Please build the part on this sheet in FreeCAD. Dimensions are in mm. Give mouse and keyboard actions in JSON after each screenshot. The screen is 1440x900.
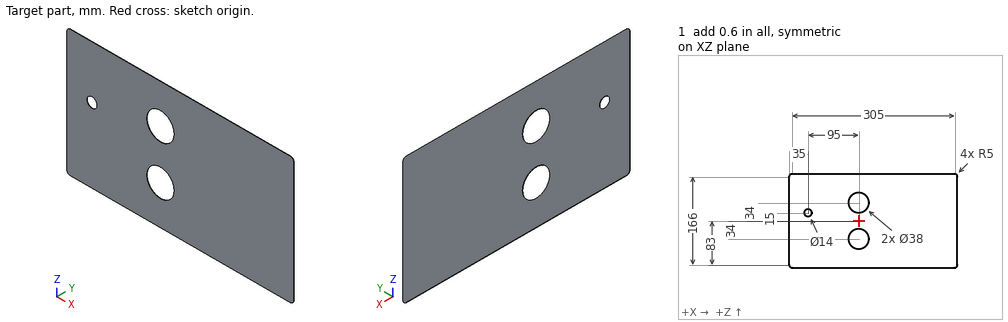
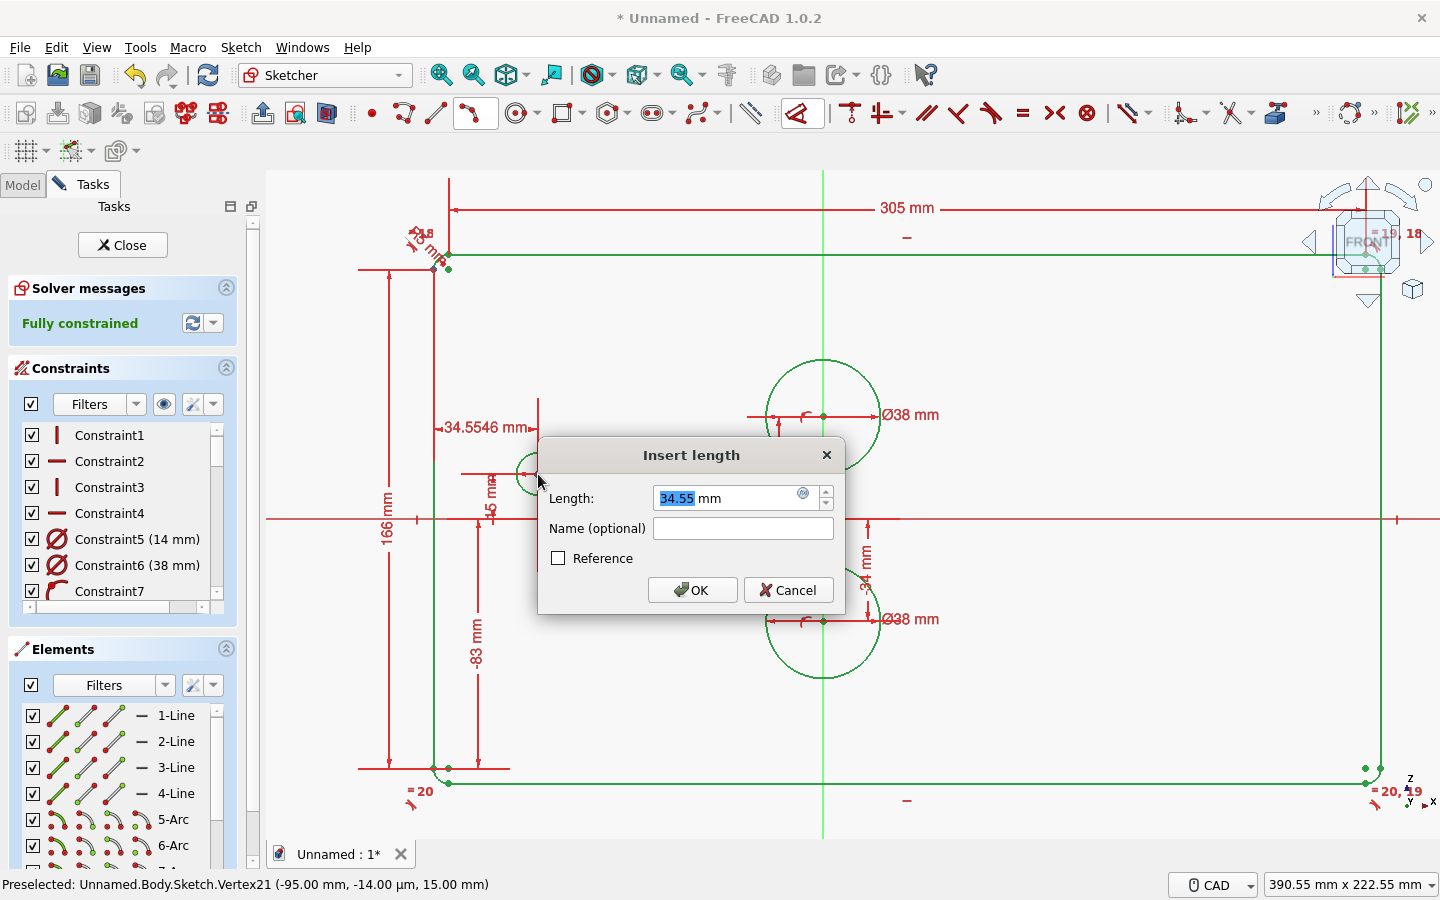
{"action": "type", "text": "35"}
{"action": "key", "text": "Return"}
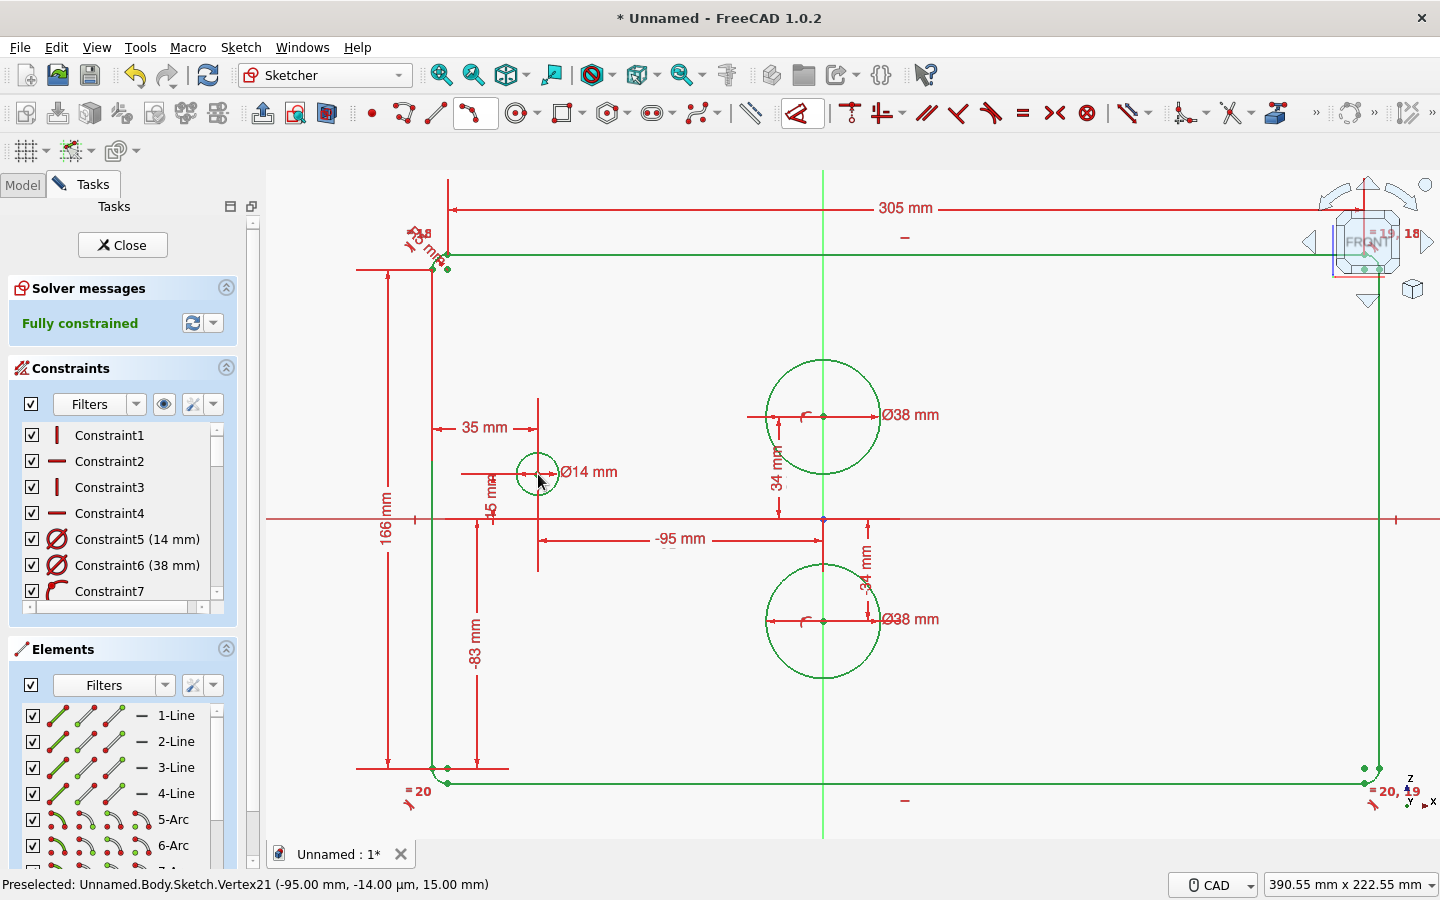
{"action": "left_click", "coordinate": [123, 245]}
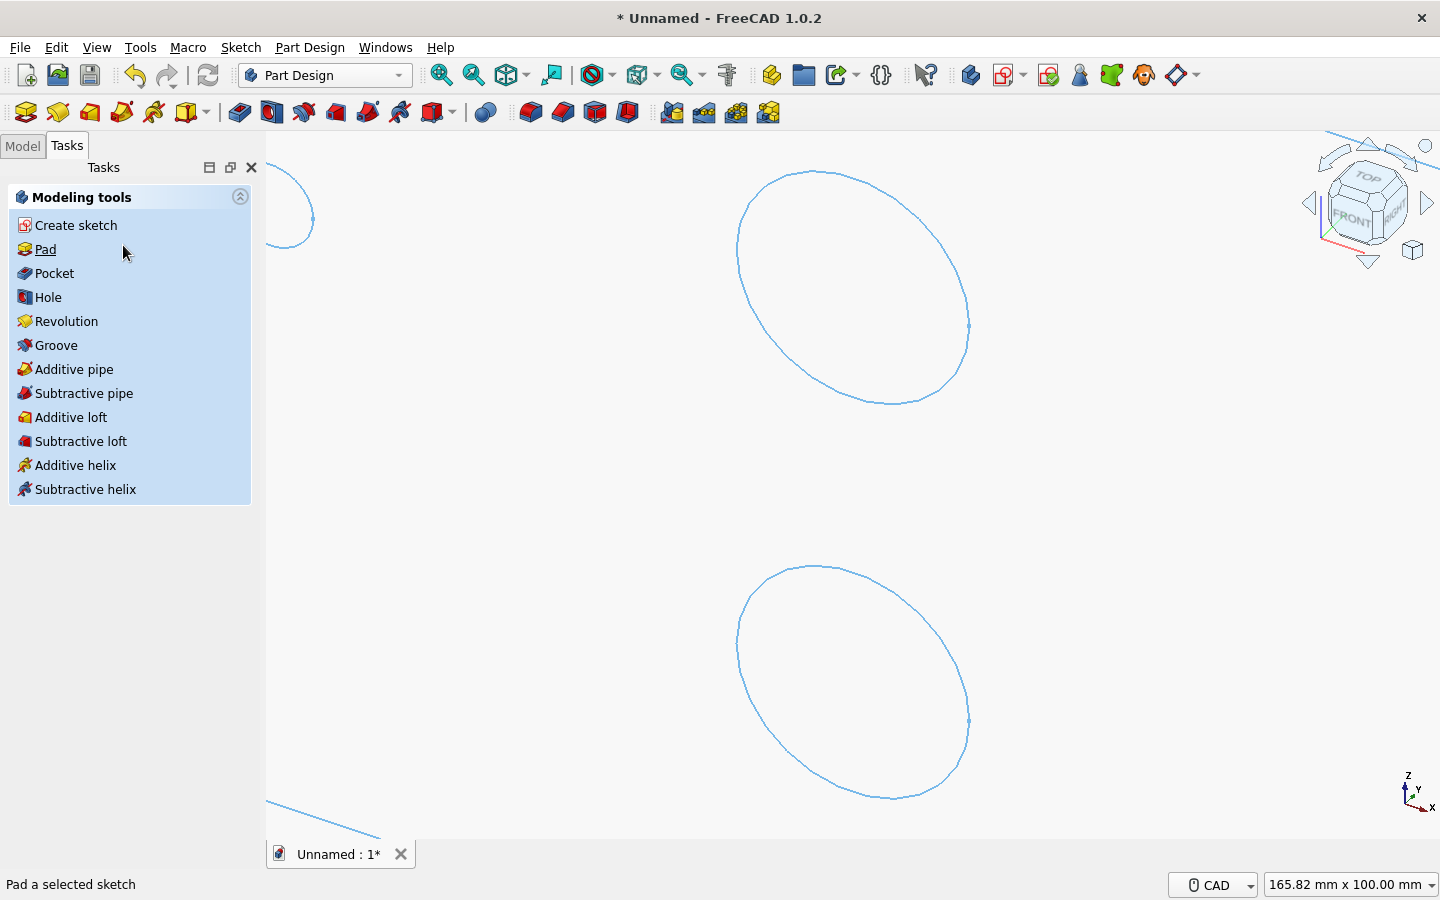
{"action": "left_click", "coordinate": [26, 112]}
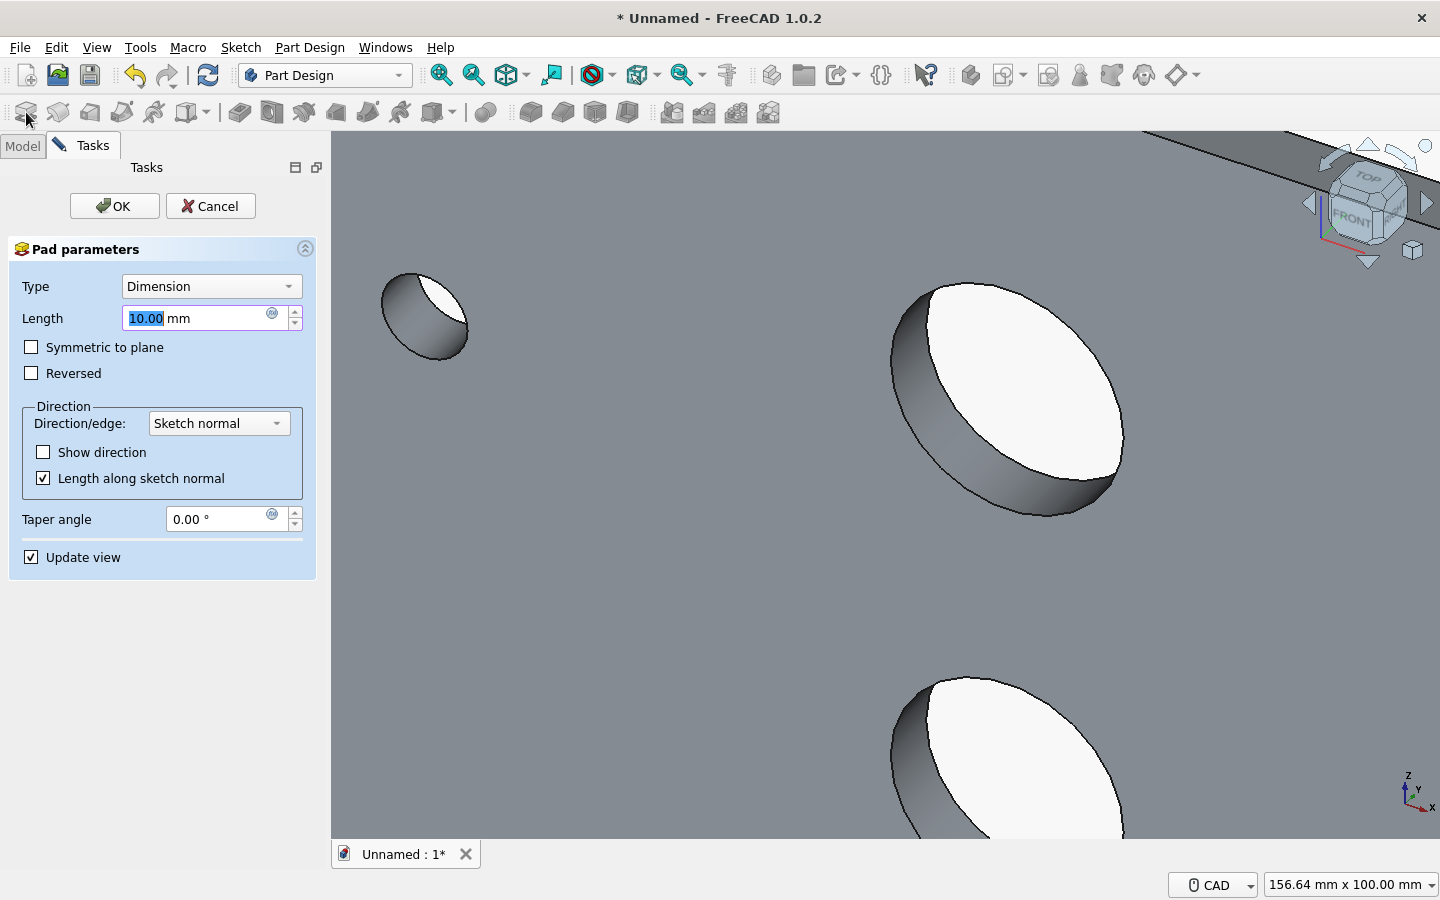
{"action": "type", "text": "0.6"}
{"action": "key", "text": "Tab"}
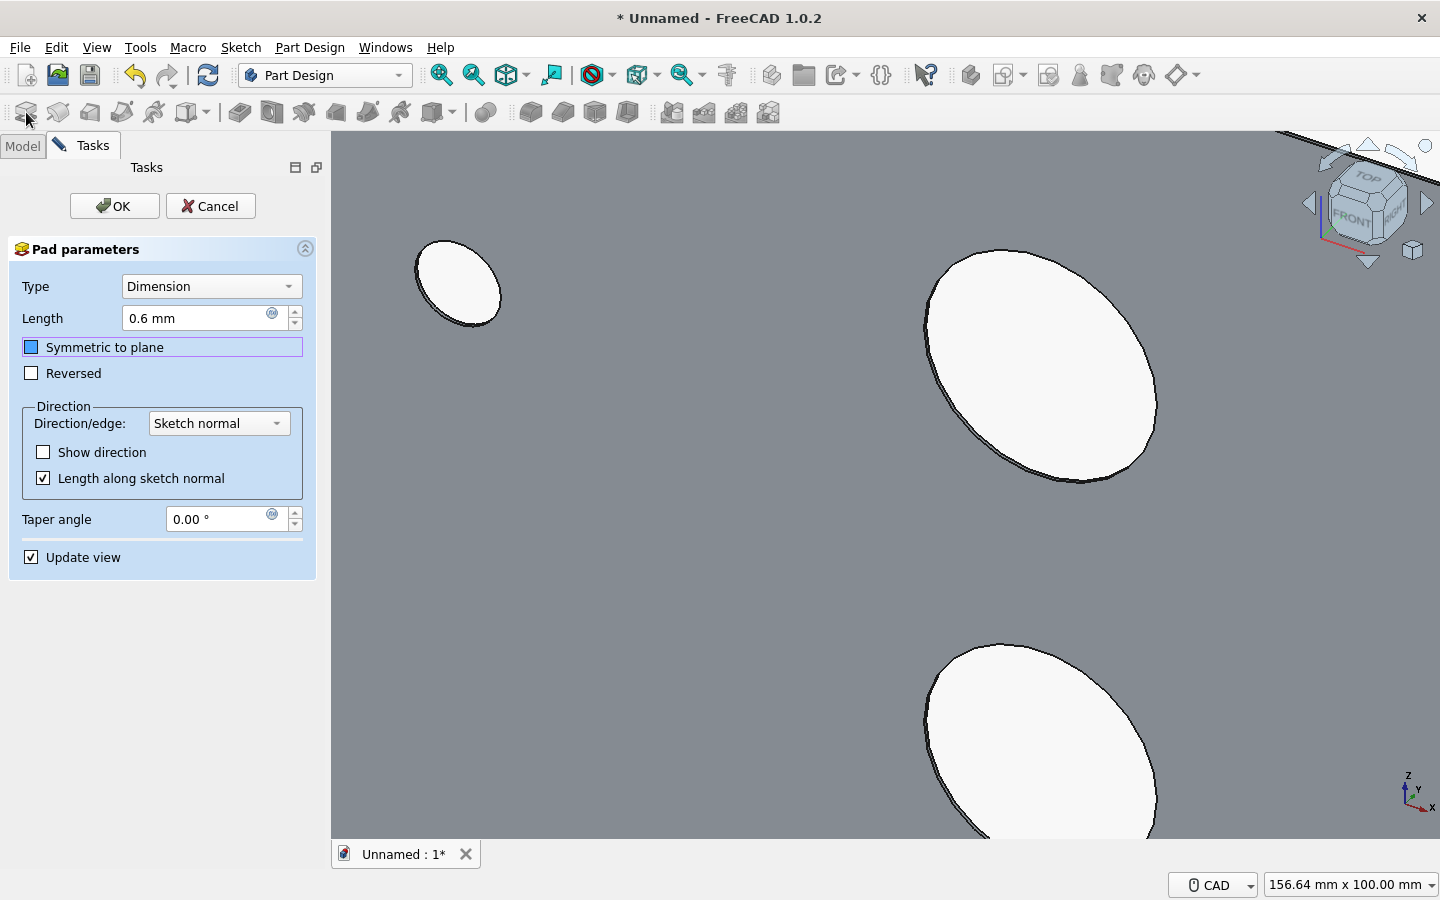
{"action": "left_click", "coordinate": [30, 347]}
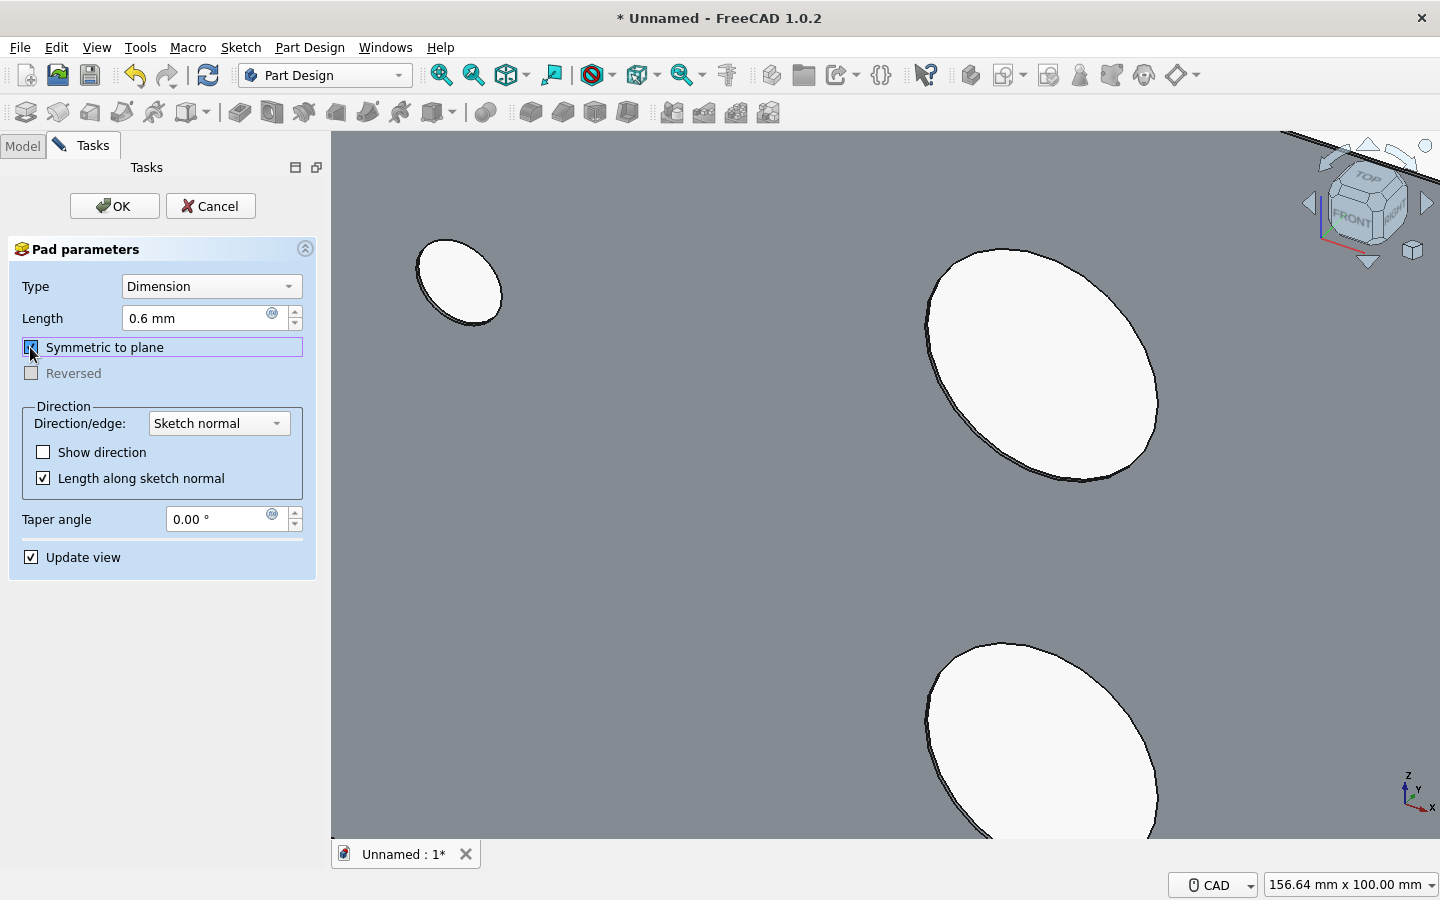
{"action": "left_click", "coordinate": [115, 206]}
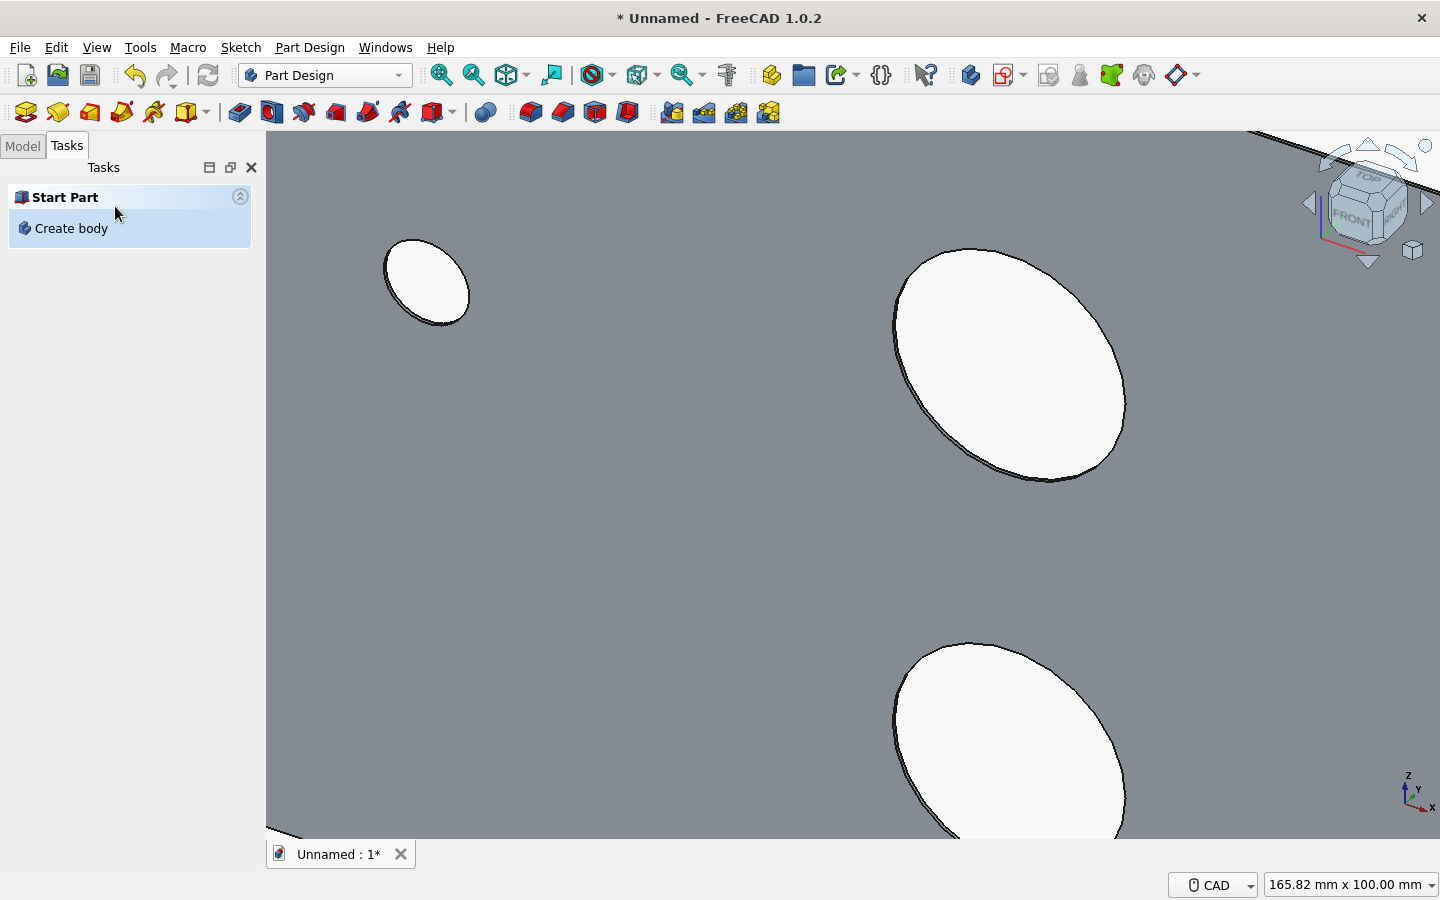
{"action": "key", "text": "0"}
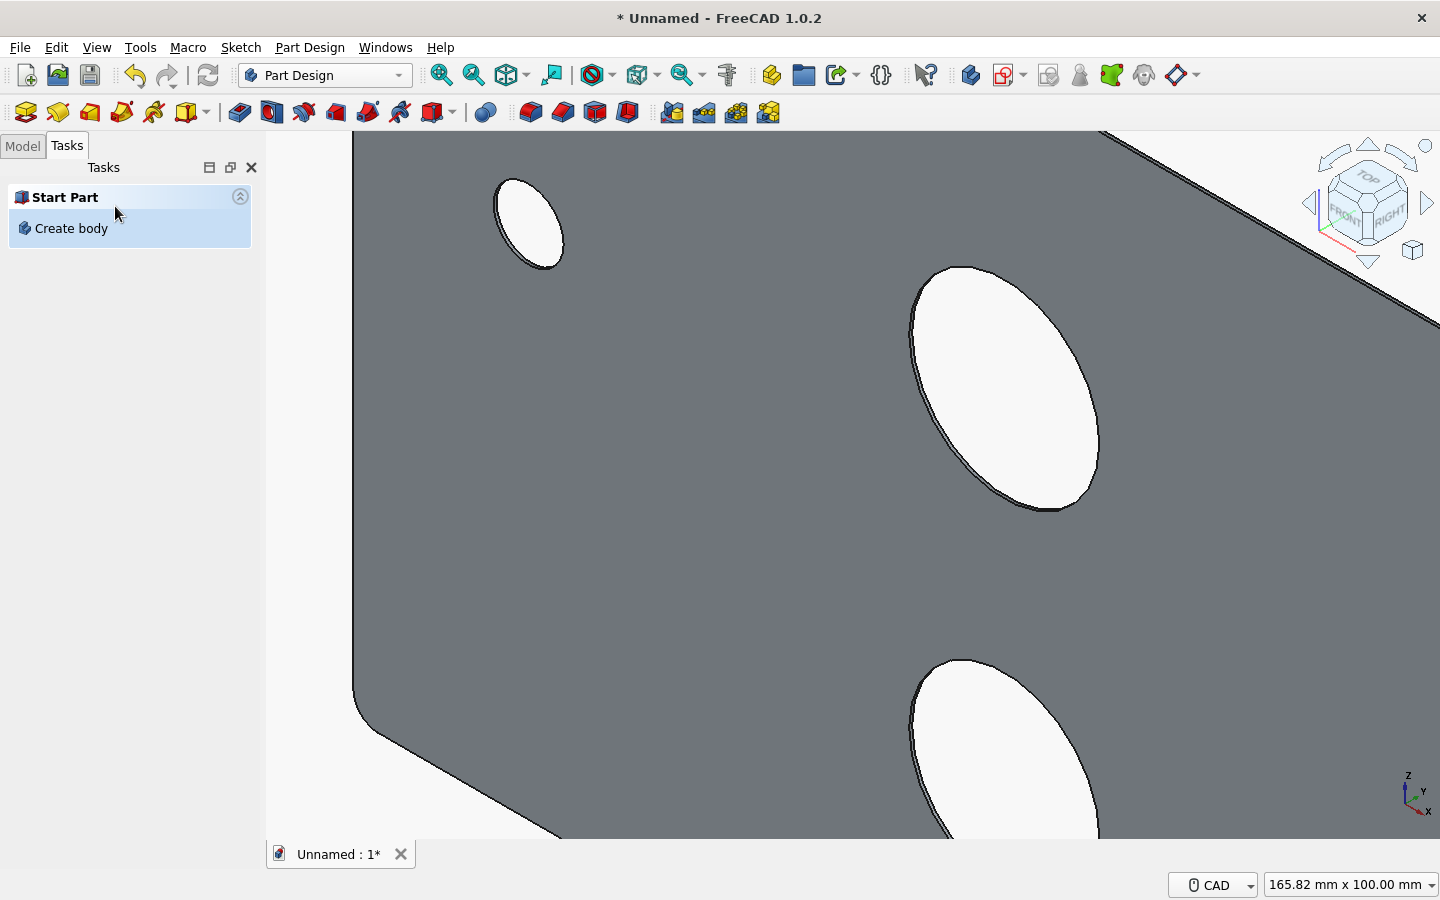
{"action": "left_click", "coordinate": [442, 76]}